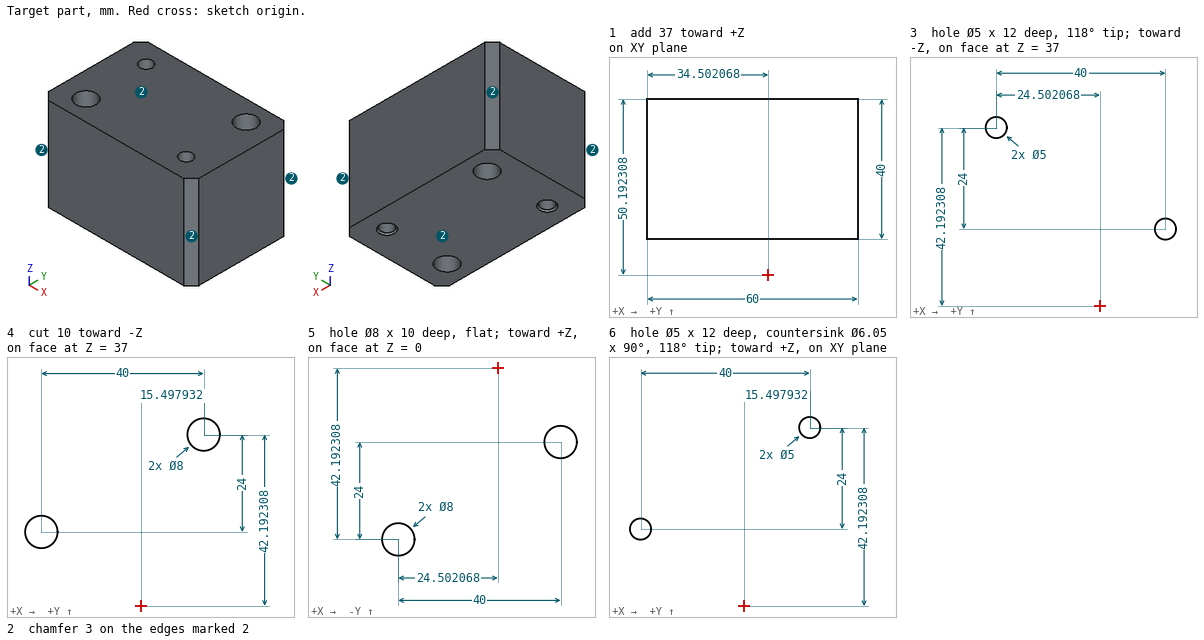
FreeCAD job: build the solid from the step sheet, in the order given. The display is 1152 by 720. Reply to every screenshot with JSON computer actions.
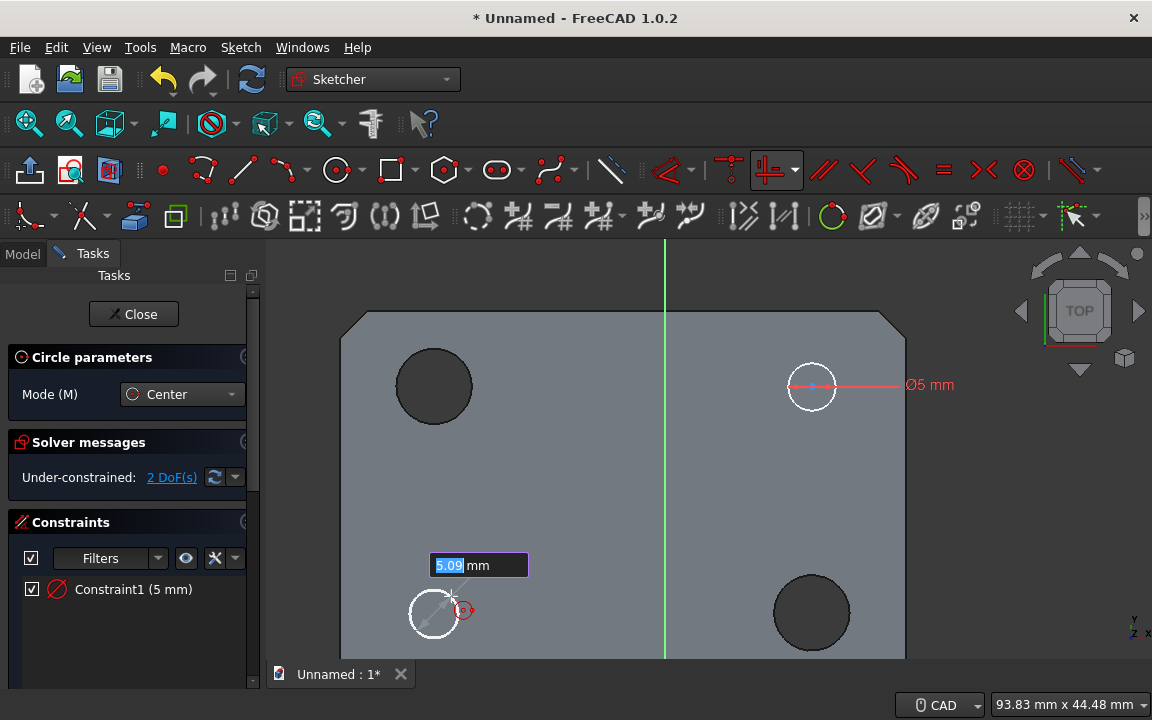
{"action": "type", "text": "5"}
{"action": "key", "text": "Return"}
{"action": "key", "text": "Escape"}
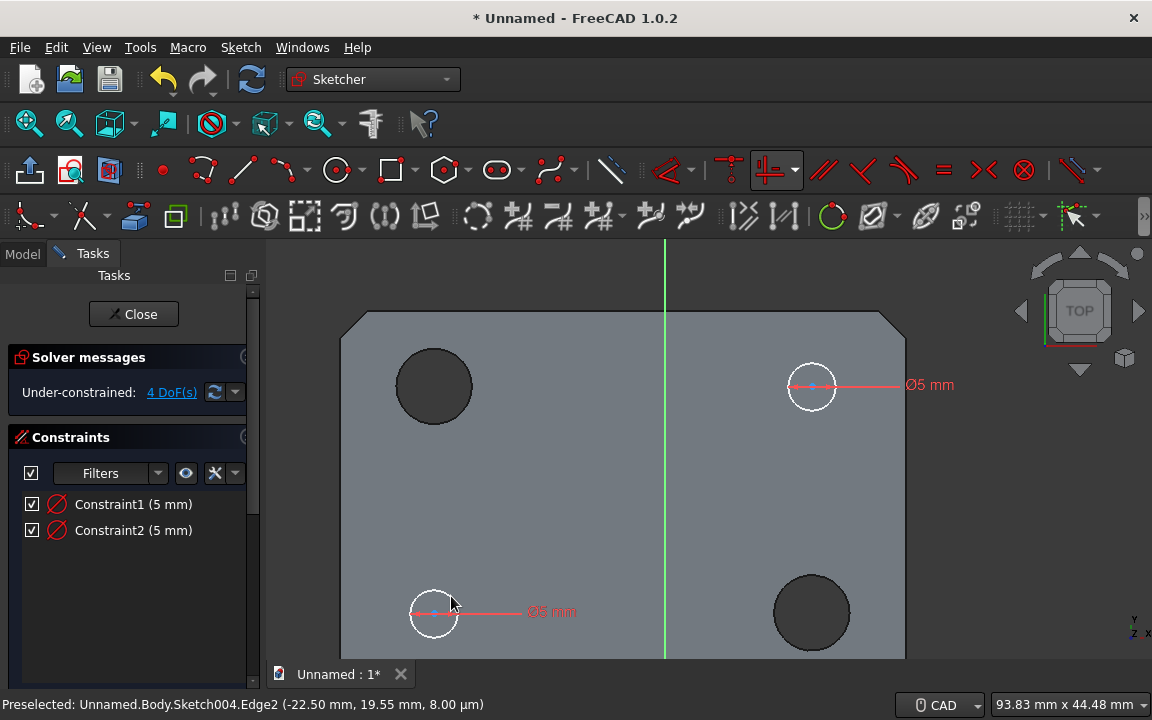
{"action": "left_click", "coordinate": [666, 170]}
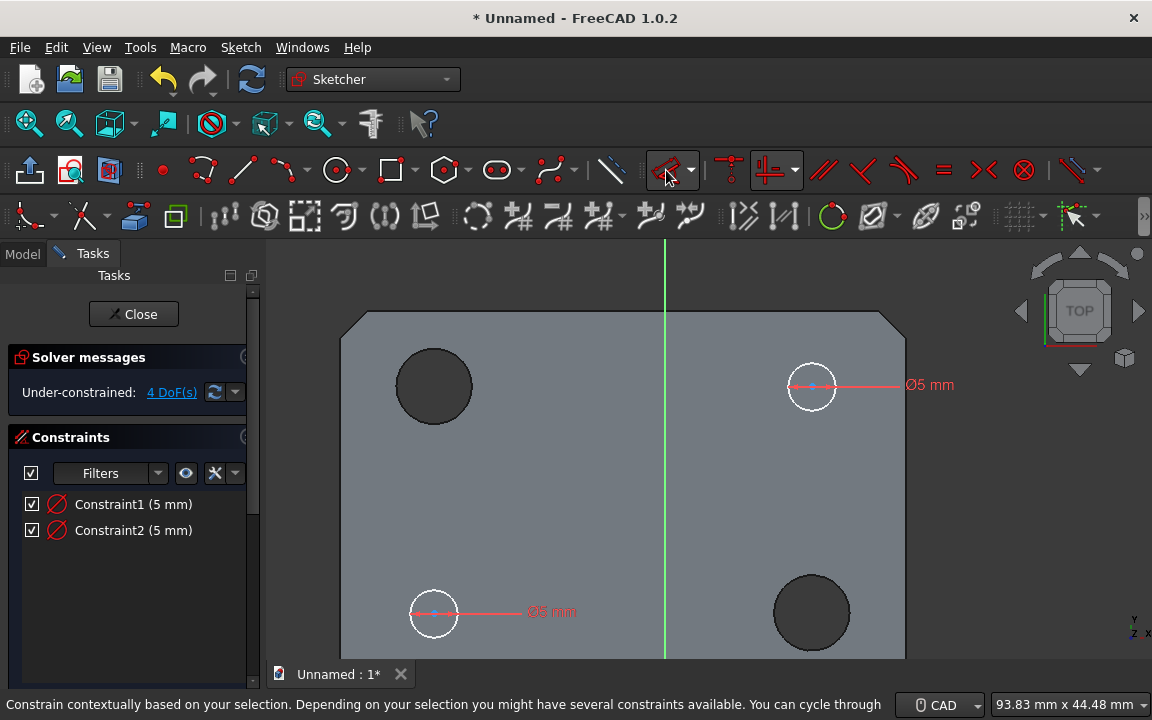
{"action": "left_click", "coordinate": [812, 387]}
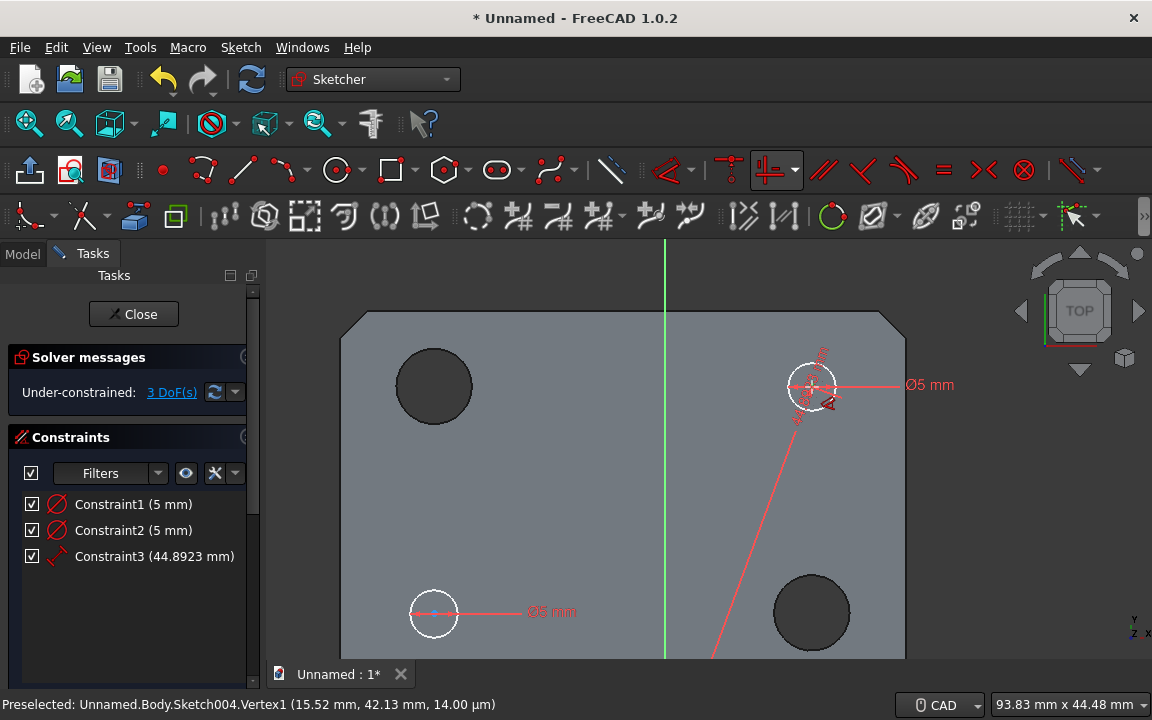
{"action": "left_click", "coordinate": [434, 614]}
{"action": "left_click", "coordinate": [623, 353]}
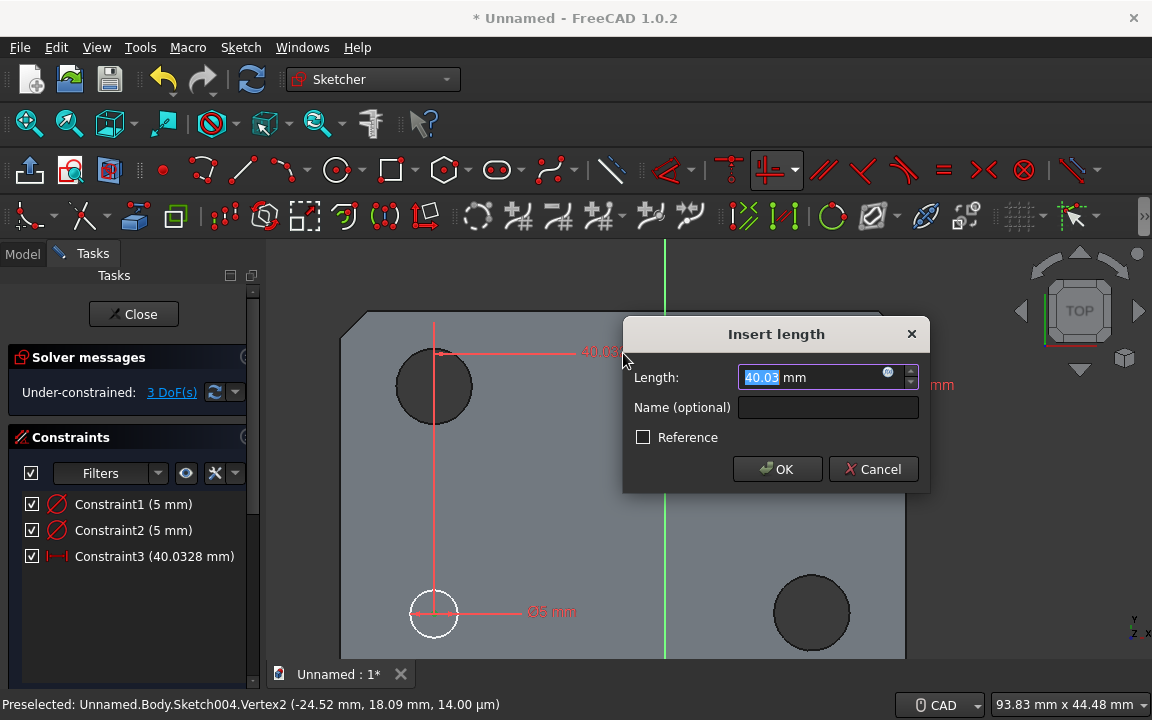
{"action": "type", "text": "40"}
{"action": "key", "text": "Return"}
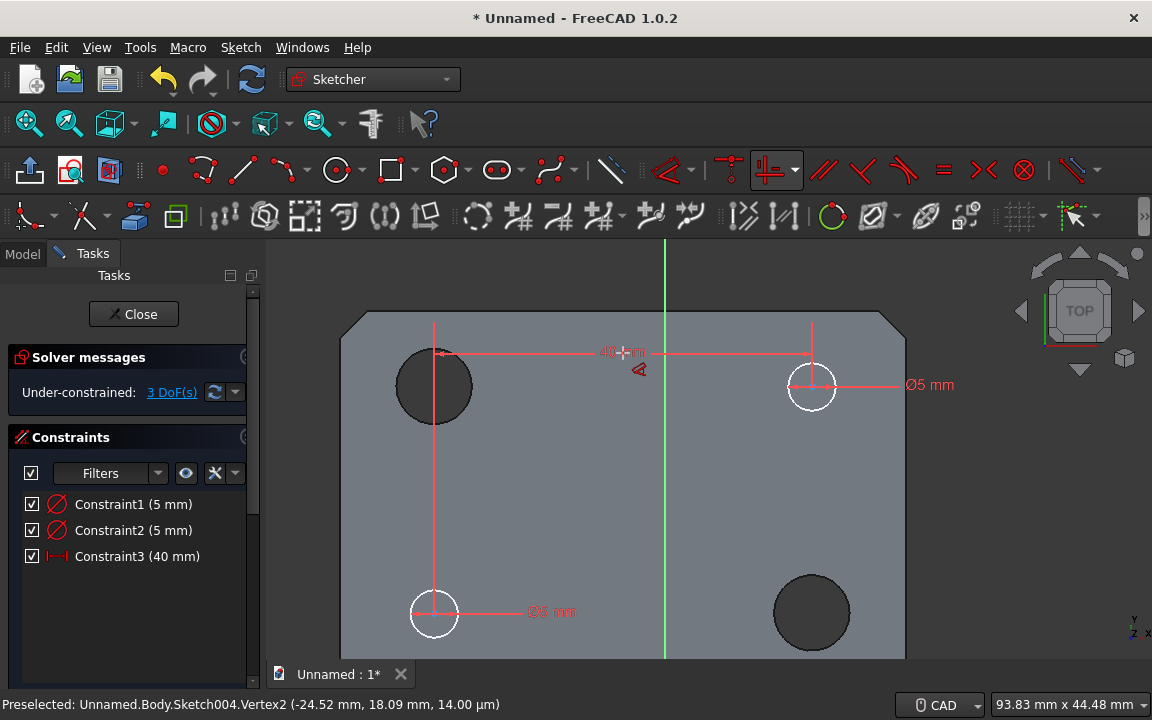
{"action": "left_click", "coordinate": [812, 387]}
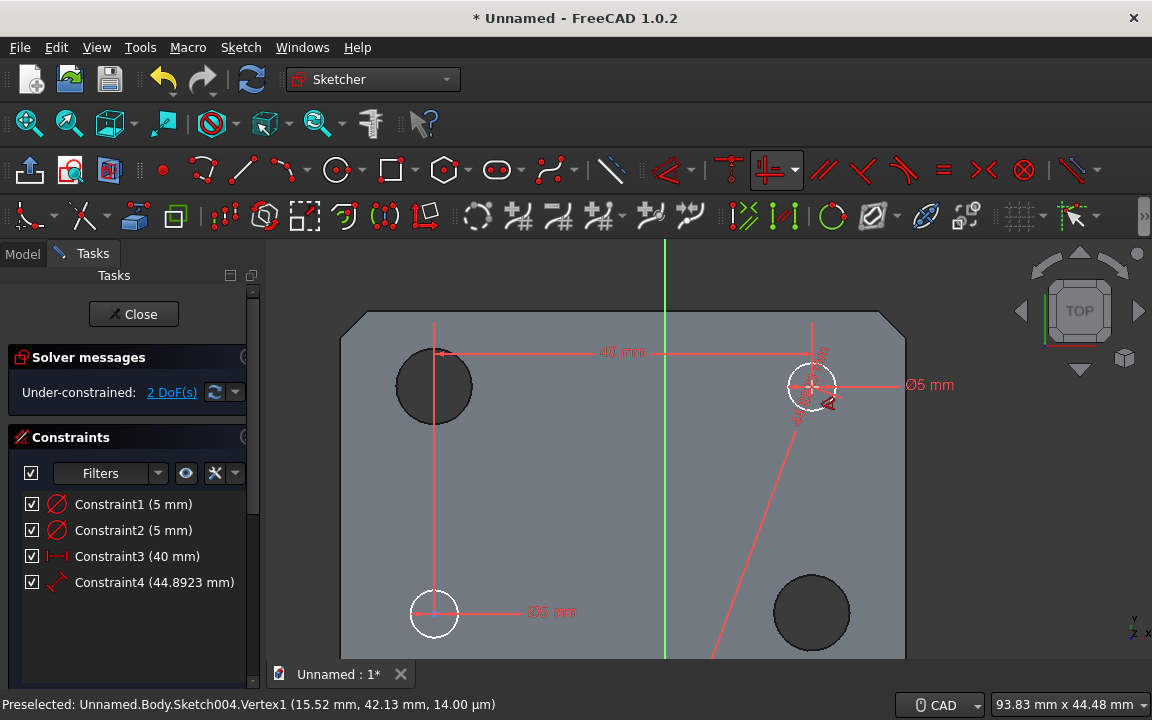
{"action": "left_click", "coordinate": [434, 614]}
{"action": "left_click", "coordinate": [846, 500]}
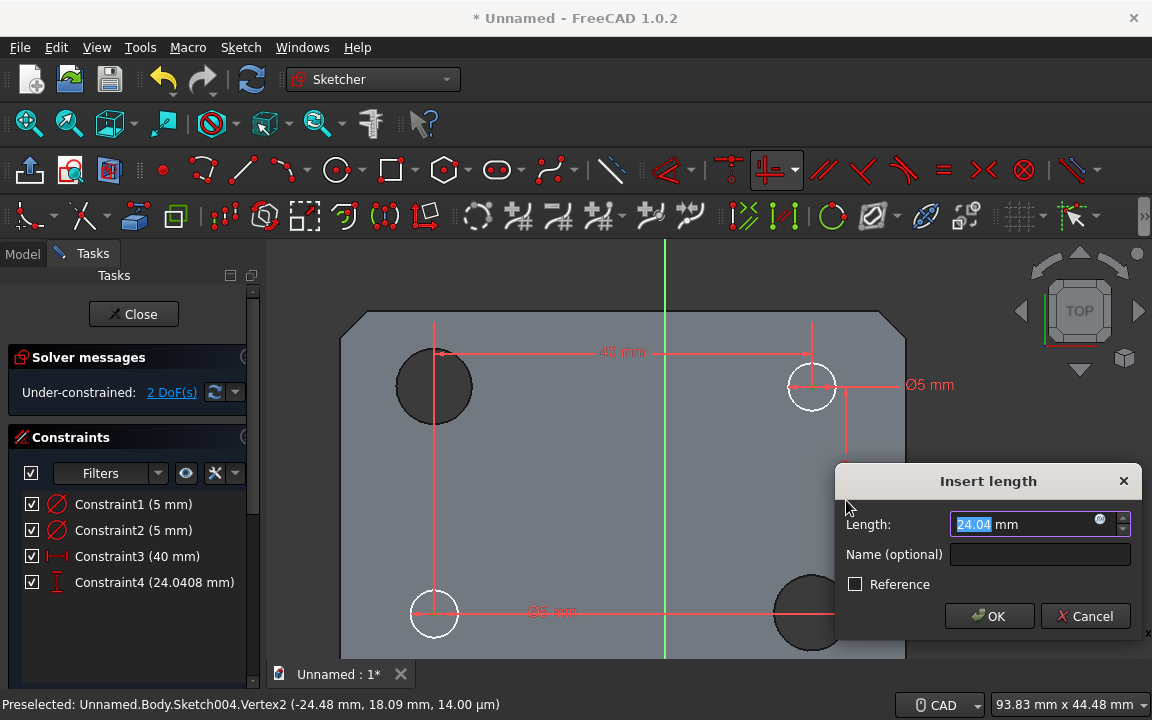
{"action": "type", "text": "24"}
{"action": "key", "text": "Return"}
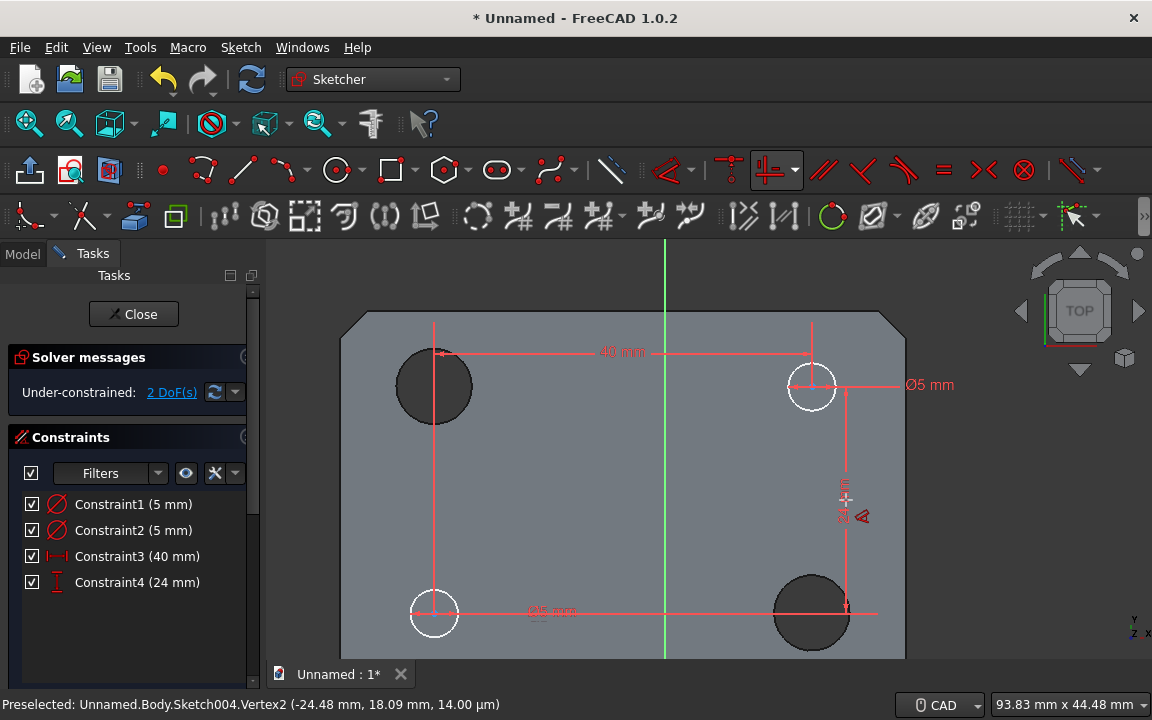
{"action": "left_click", "coordinate": [812, 387]}
{"action": "left_click", "coordinate": [739, 353]}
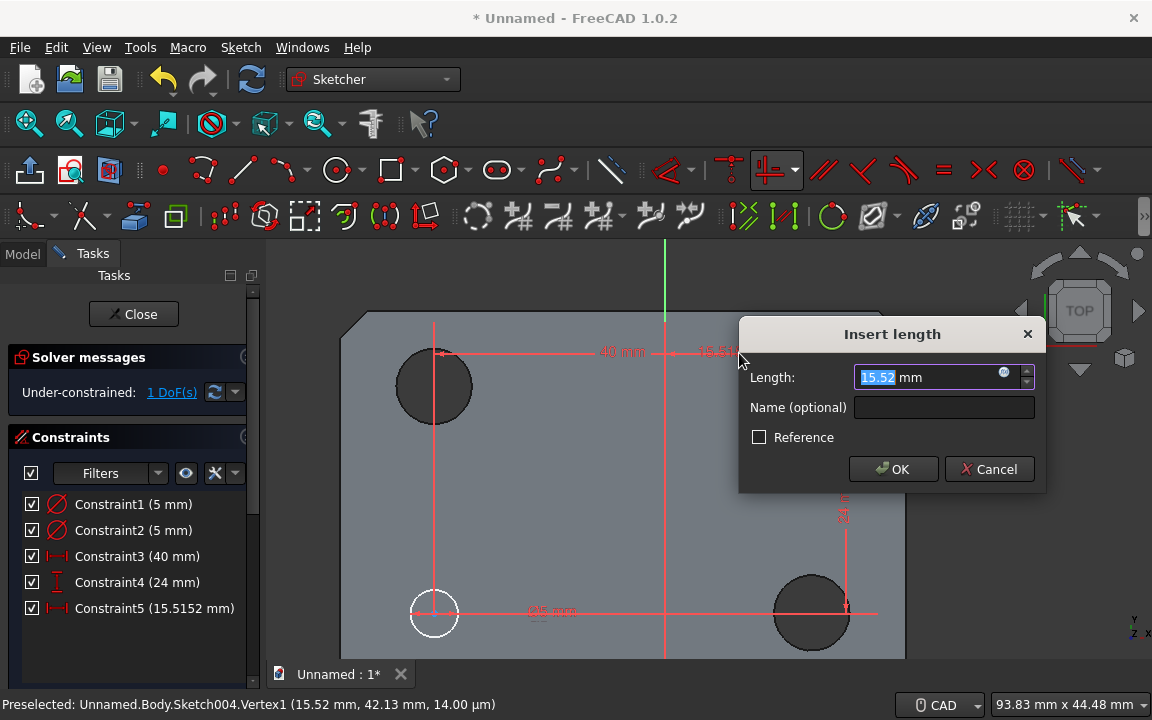
{"action": "type", "text": "15.497932"}
{"action": "key", "text": "Return"}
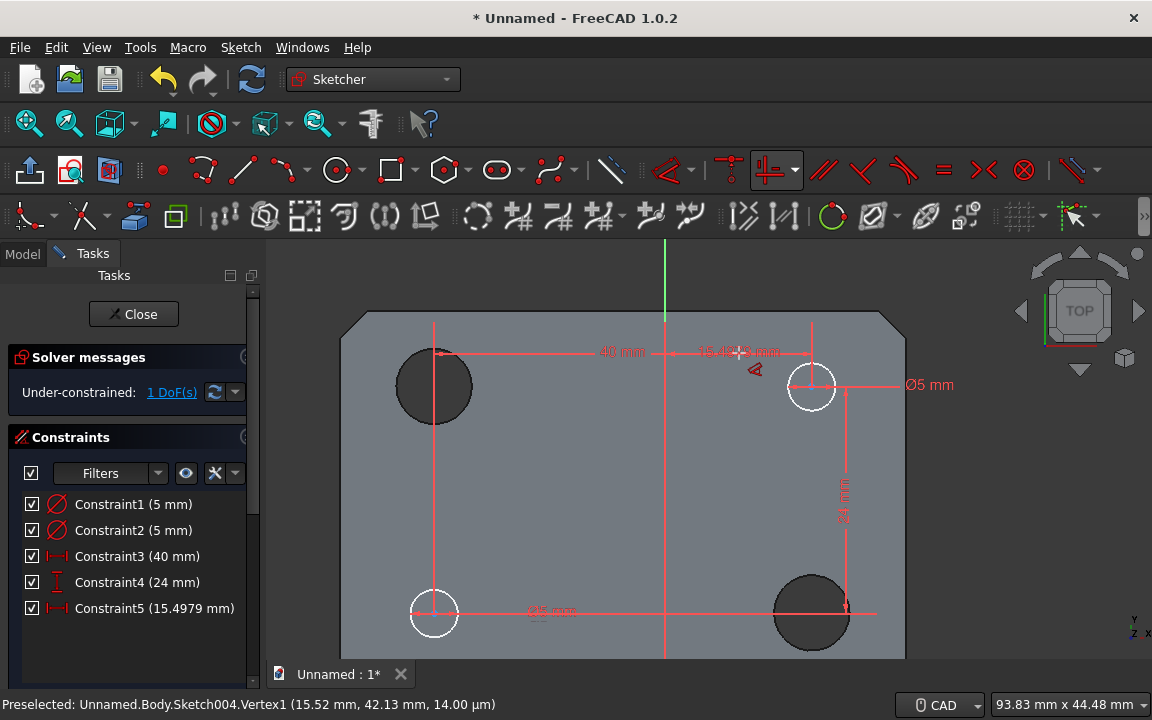
{"action": "left_click", "coordinate": [812, 387]}
{"action": "left_click", "coordinate": [846, 453]}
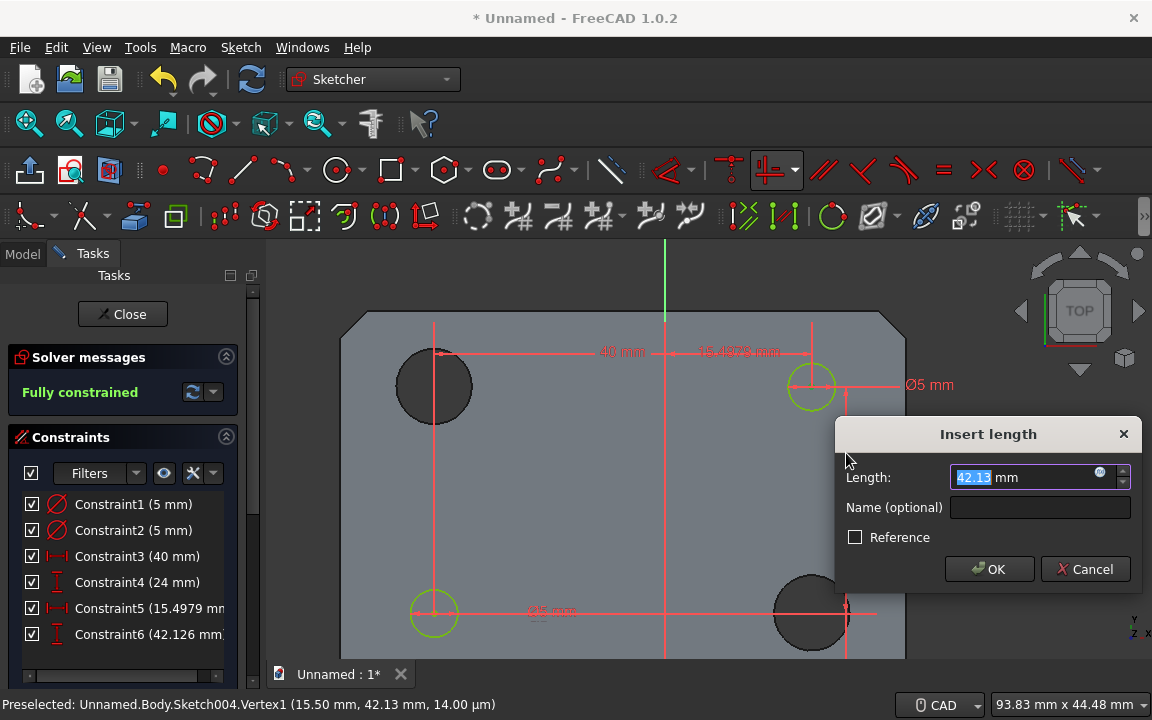
{"action": "type", "text": "42.192308"}
{"action": "key", "text": "Return"}
{"action": "key", "text": "Escape"}